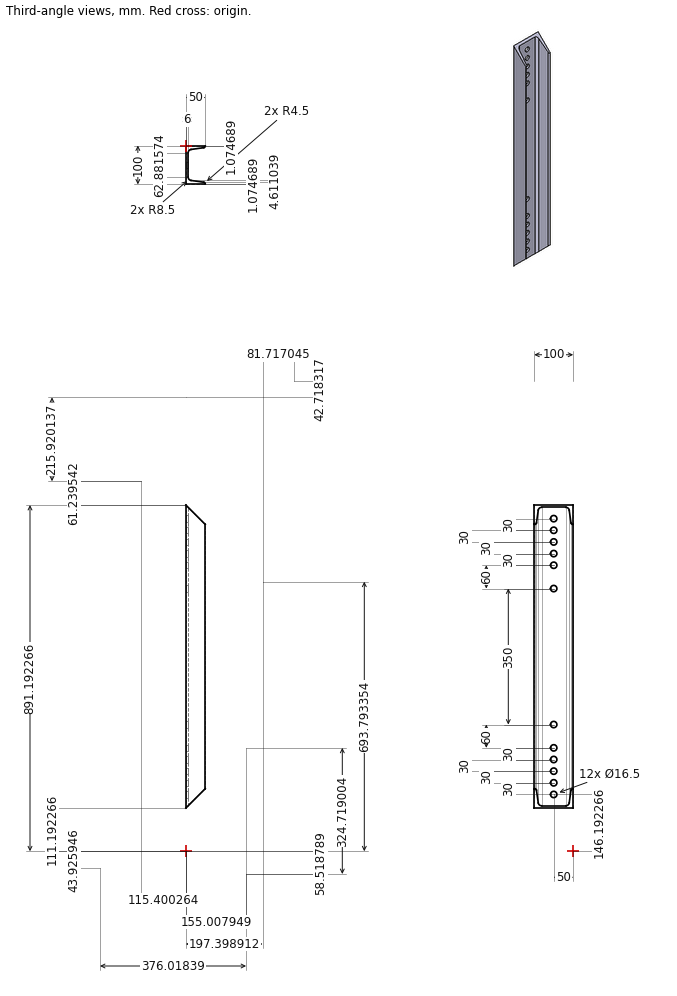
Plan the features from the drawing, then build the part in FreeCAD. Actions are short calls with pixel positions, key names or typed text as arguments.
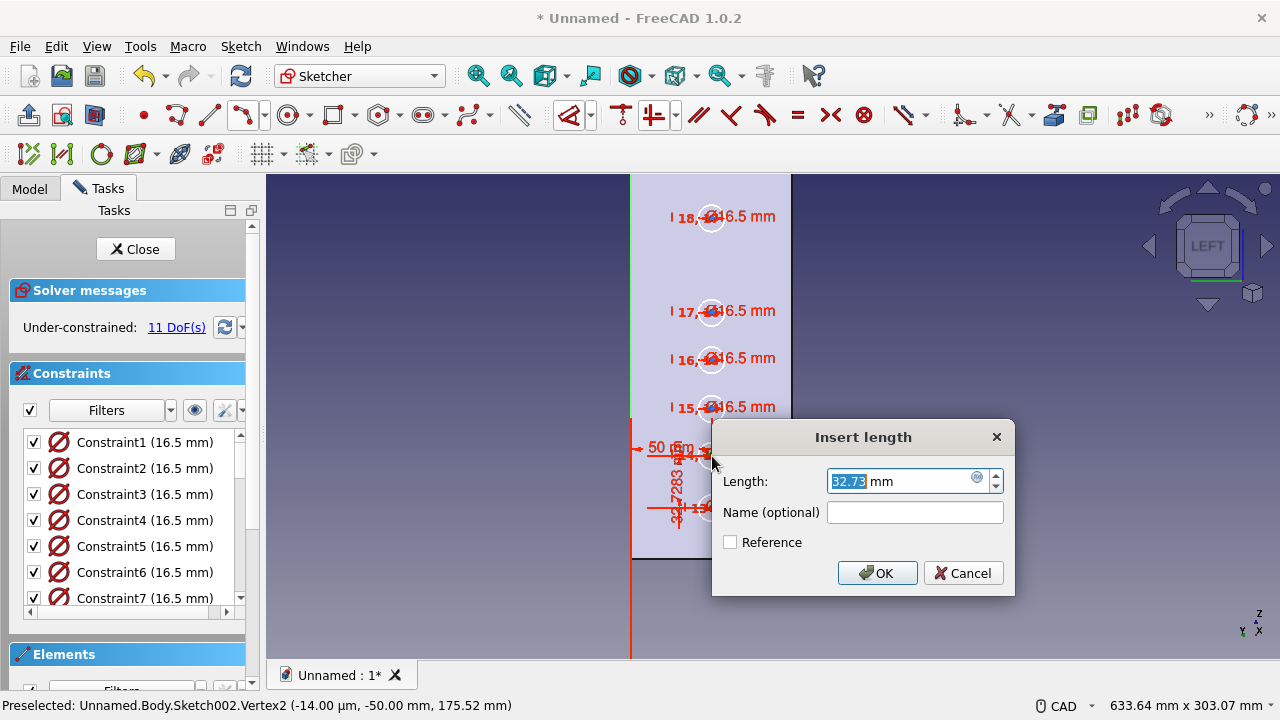
text(30)
key(Return)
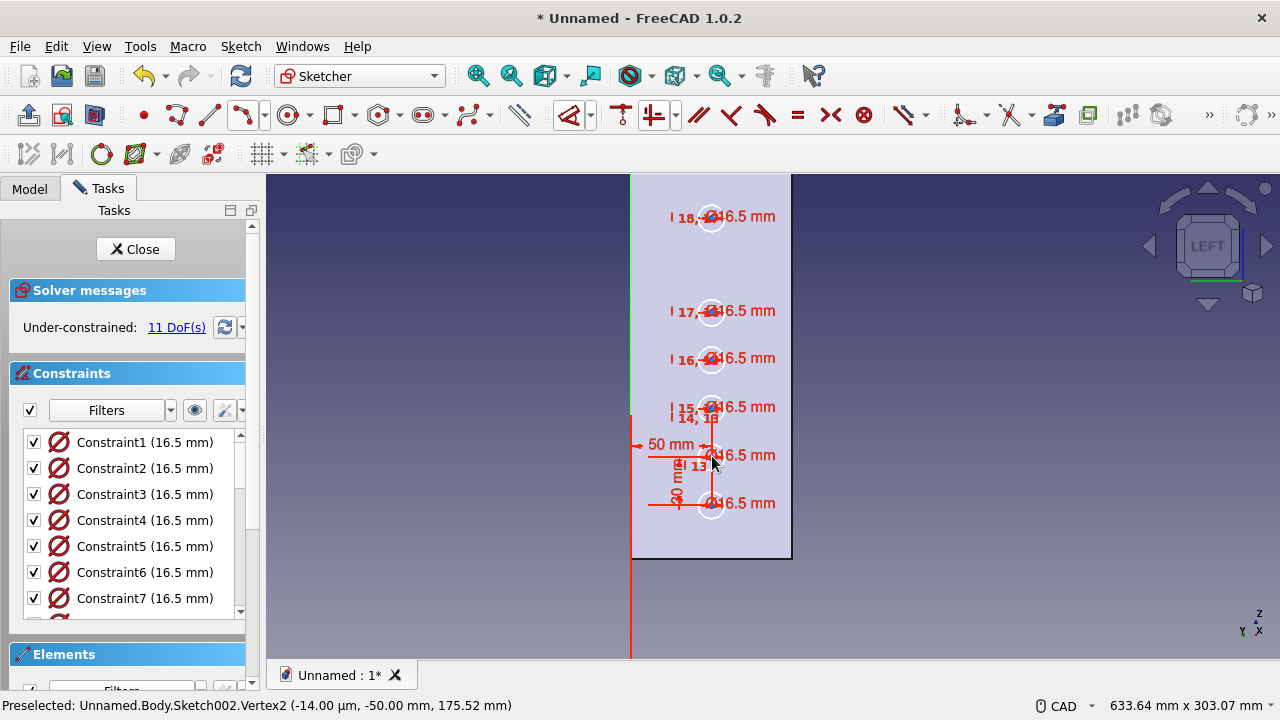
click(712, 457)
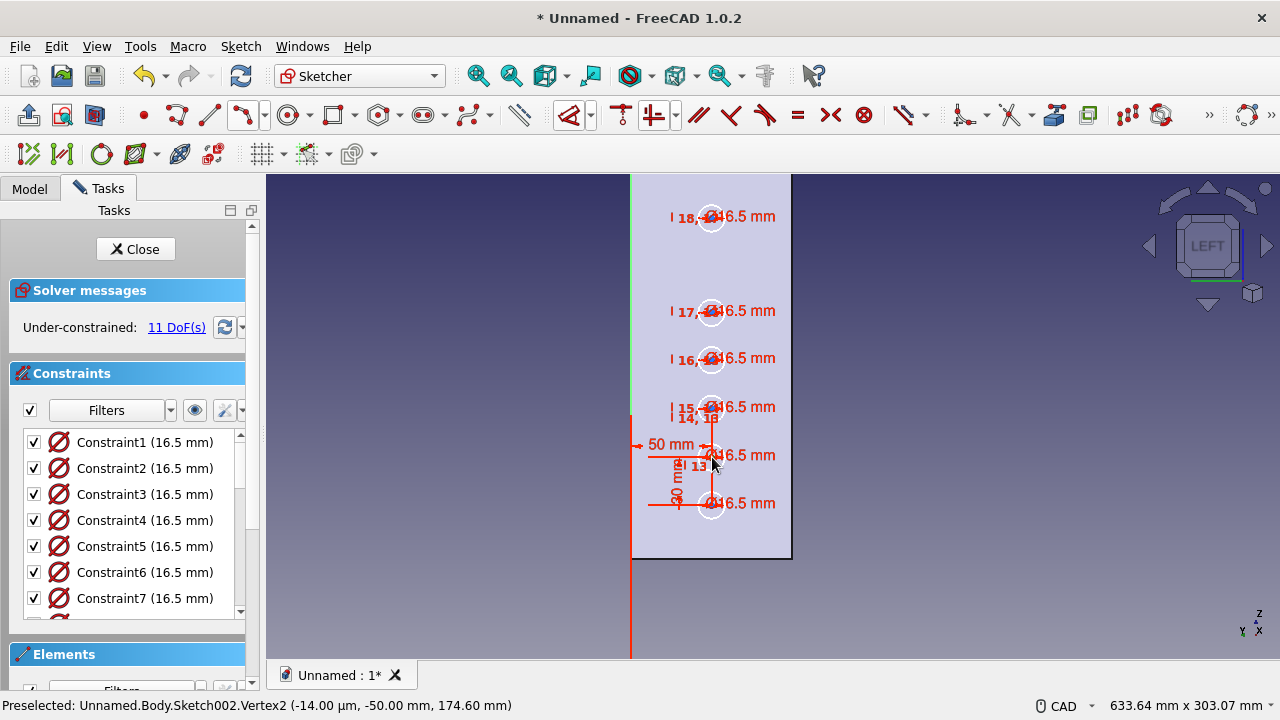
click(712, 409)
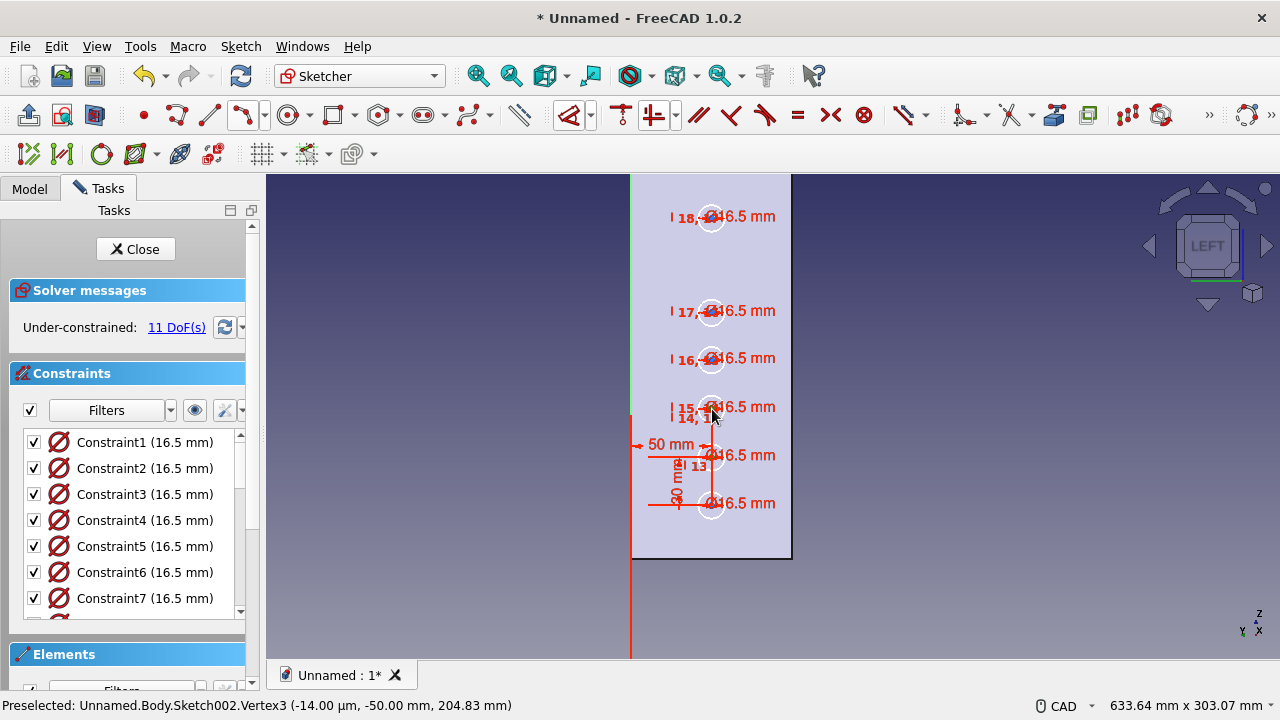
click(590, 116)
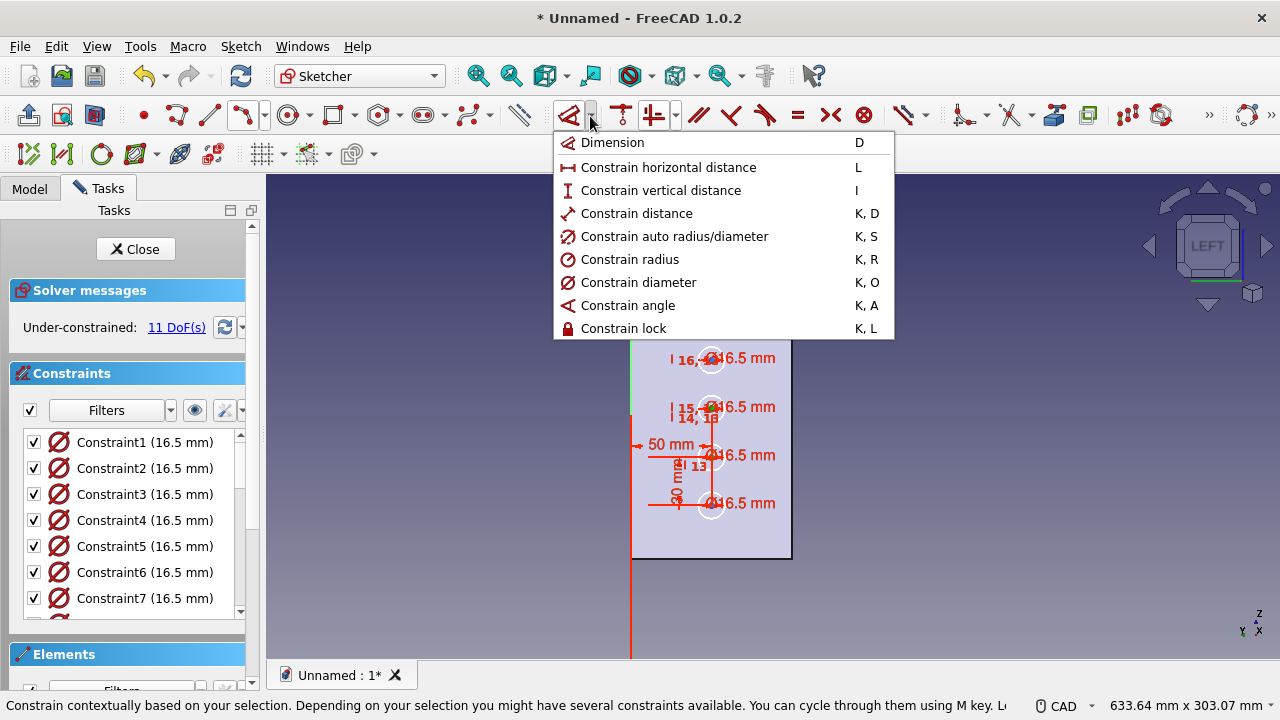
click(724, 190)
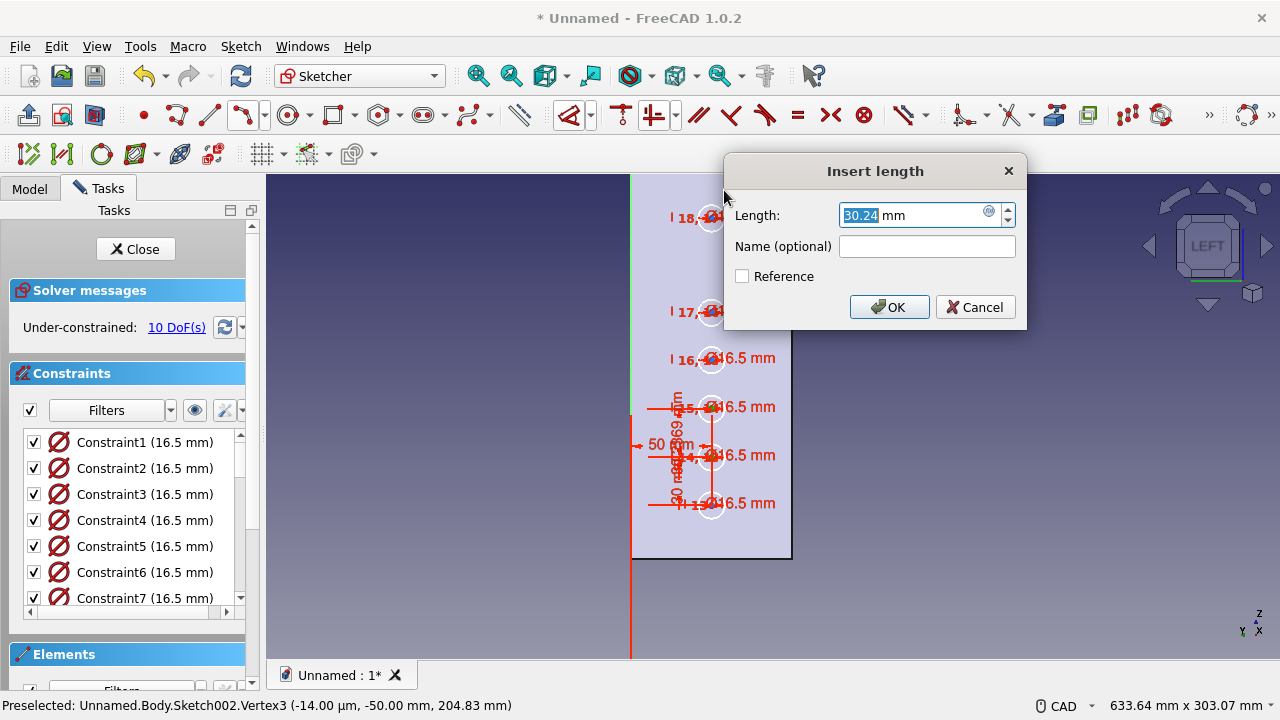
text(30)
key(Return)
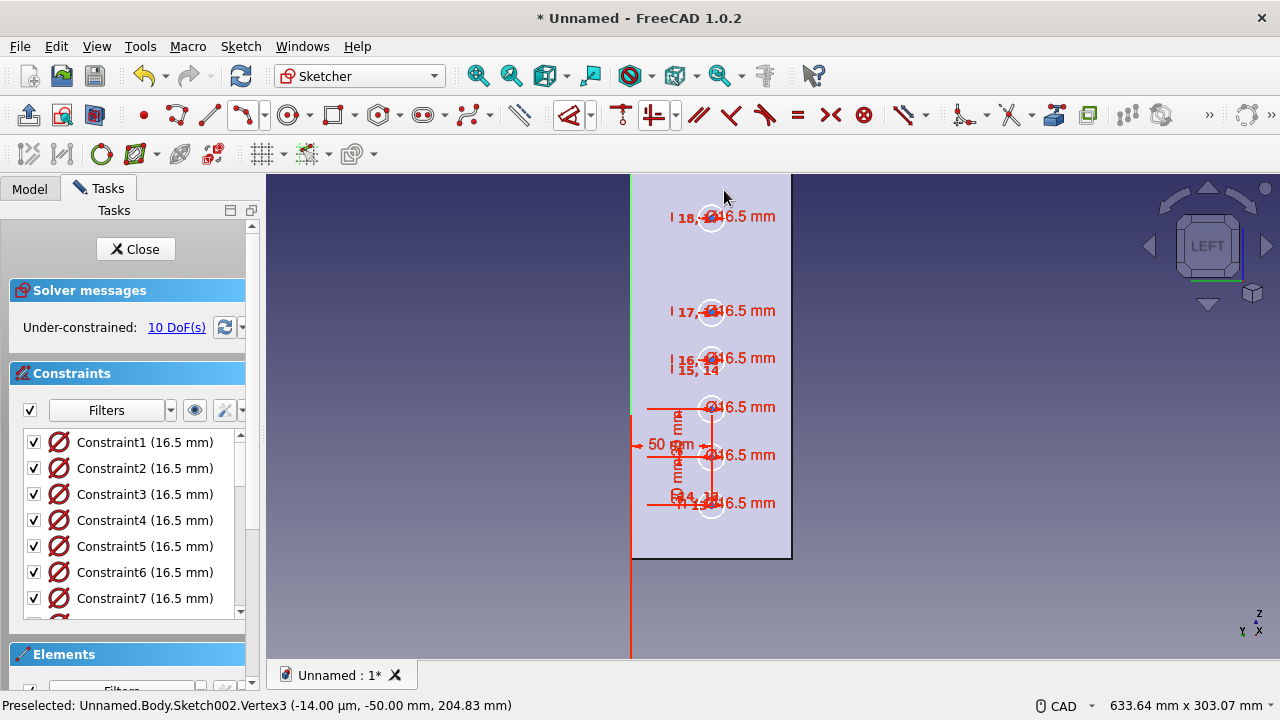
click(712, 409)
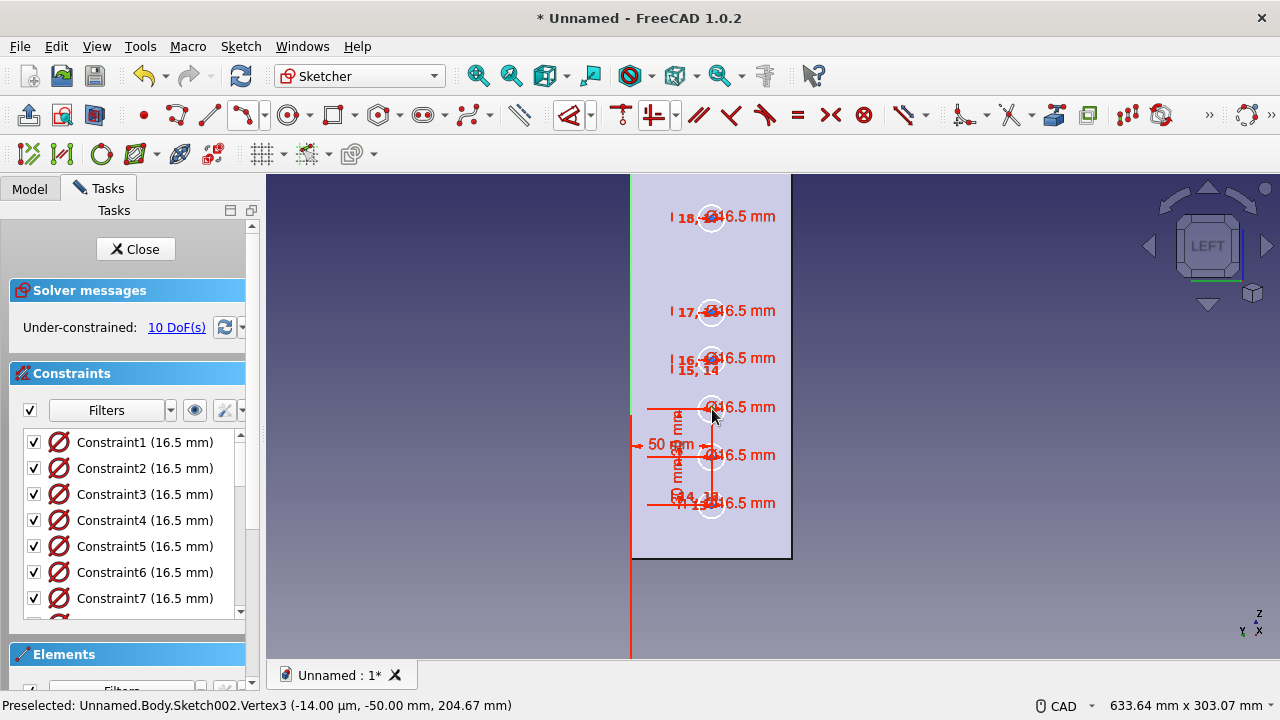
click(712, 360)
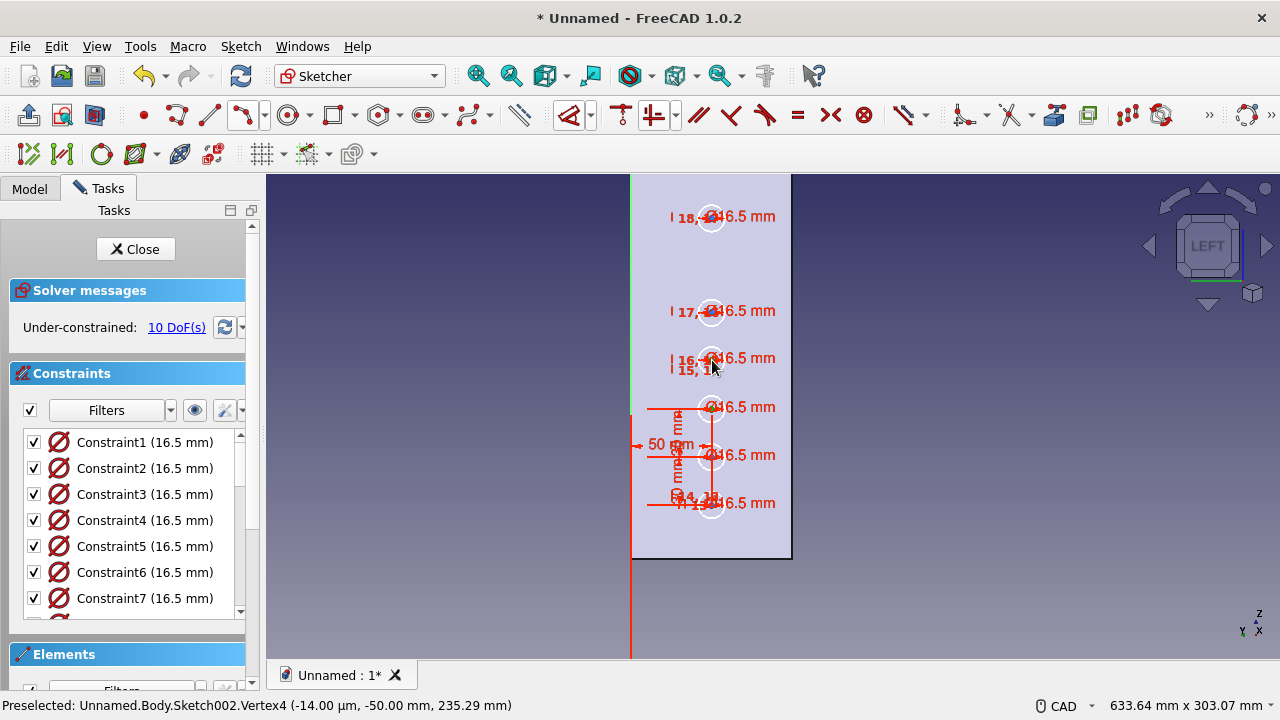
click(590, 116)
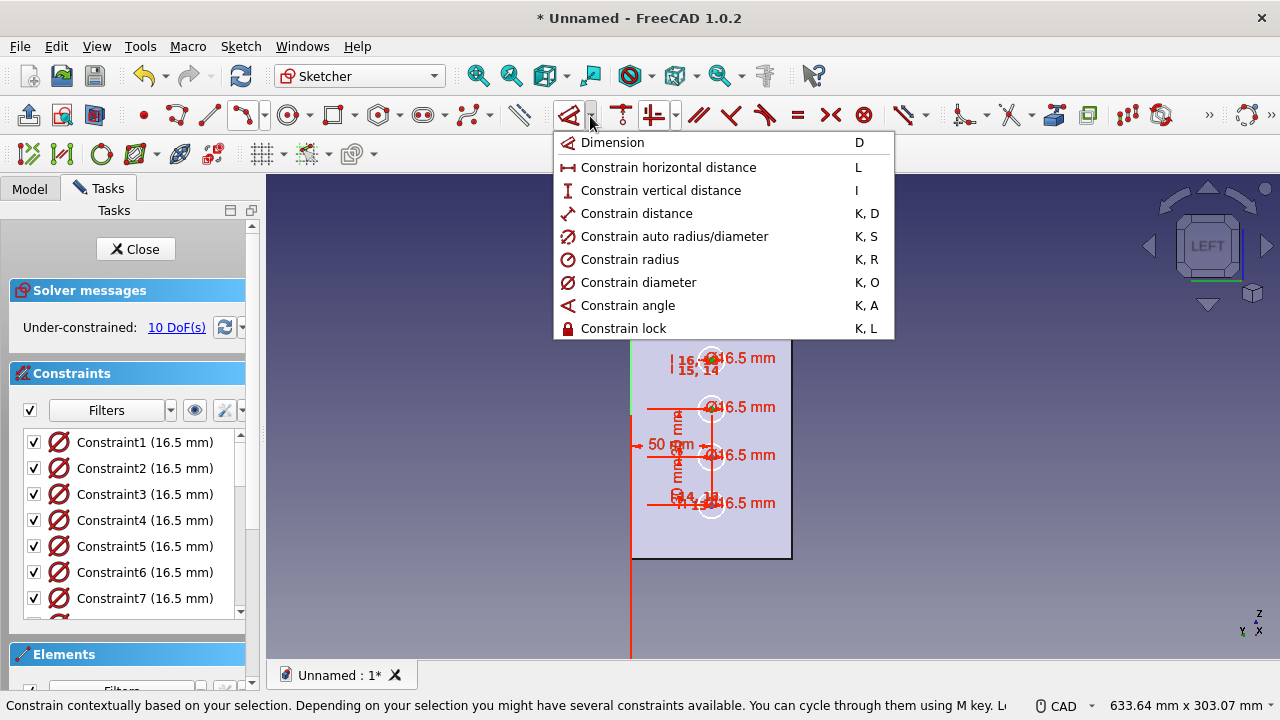
click(724, 190)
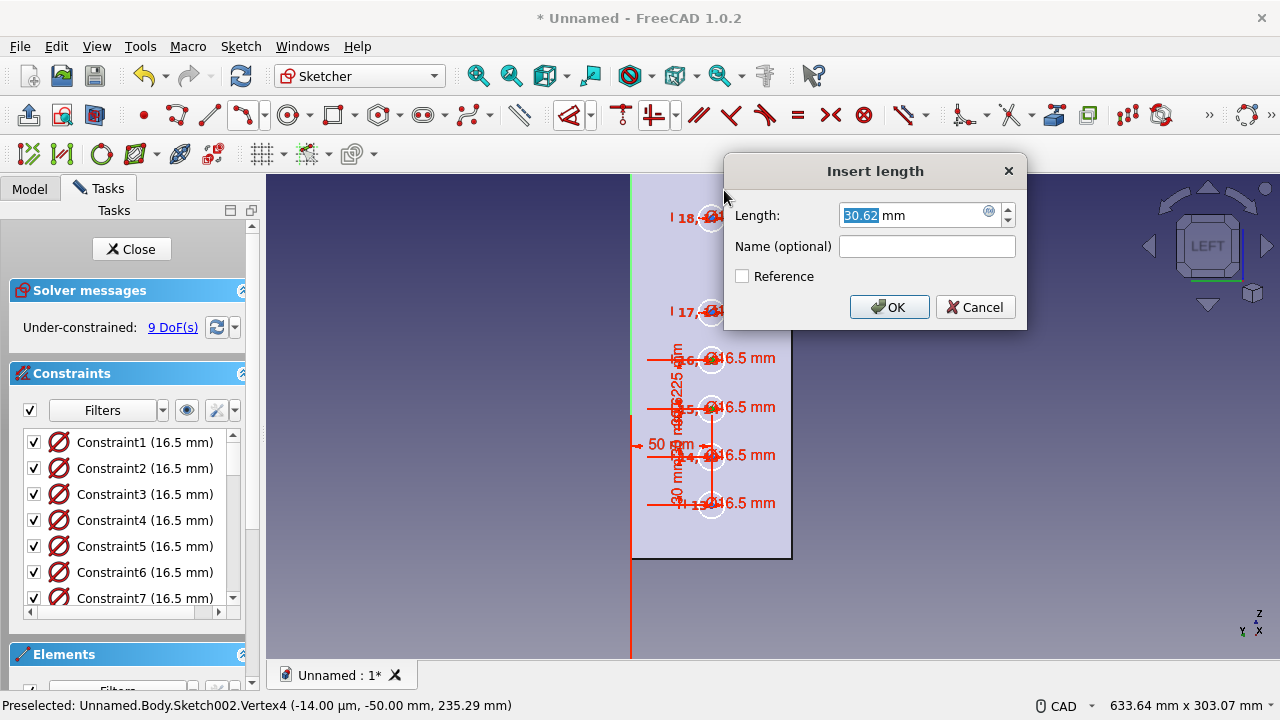
text(30)
key(Return)